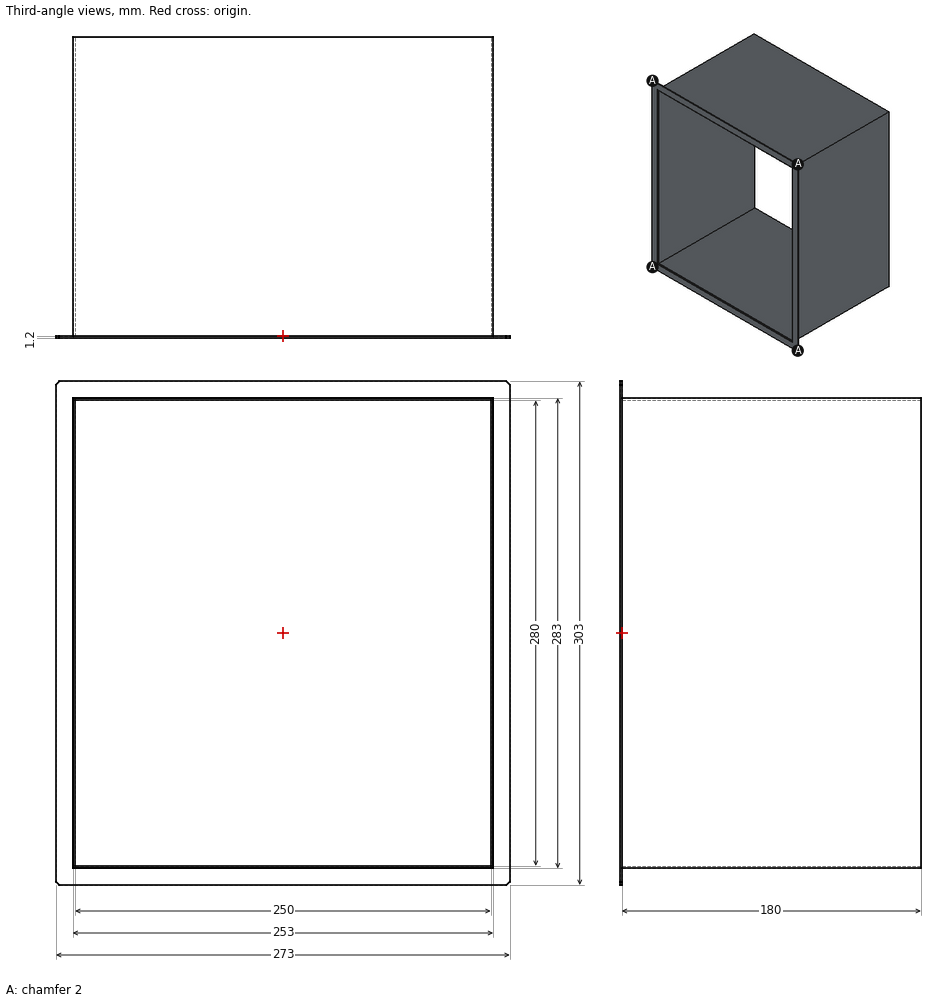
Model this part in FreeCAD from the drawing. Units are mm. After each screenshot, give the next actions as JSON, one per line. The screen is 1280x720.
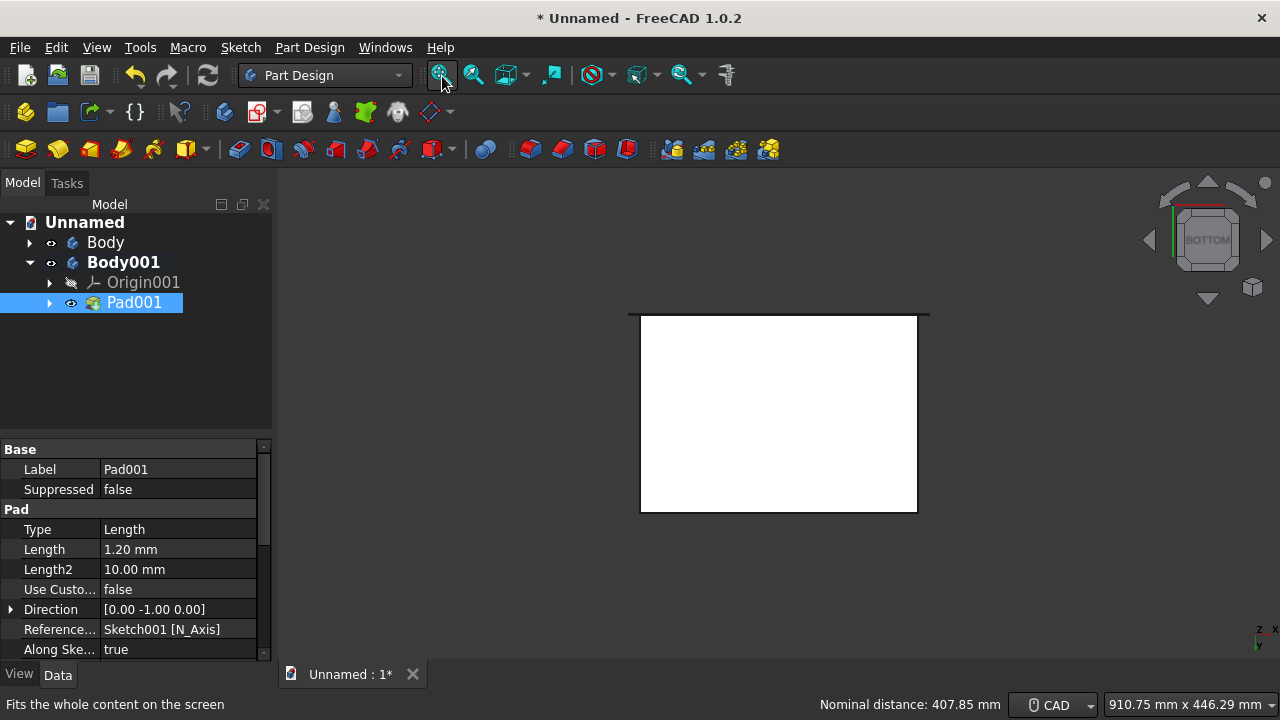
{"action": "scroll", "coordinate": [629, 313], "scroll_direction": "up", "scroll_amount": 15}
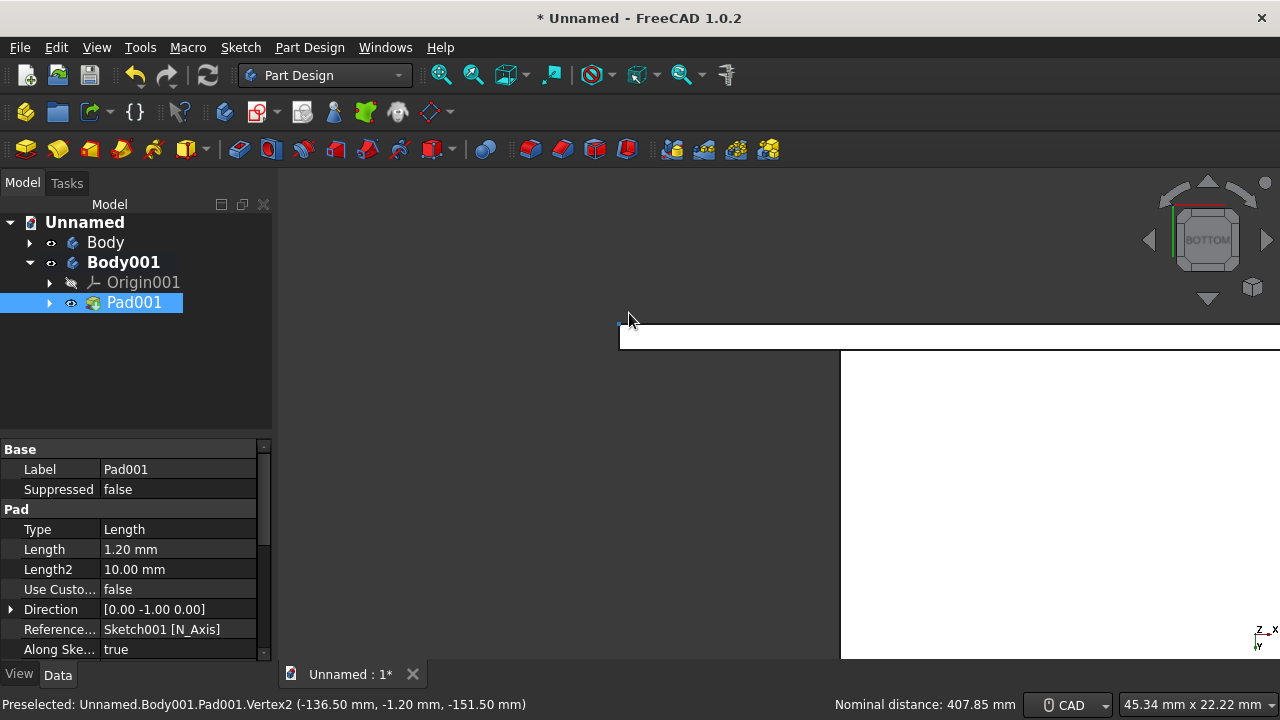
{"action": "left_click", "coordinate": [619, 336], "text": "ctrl"}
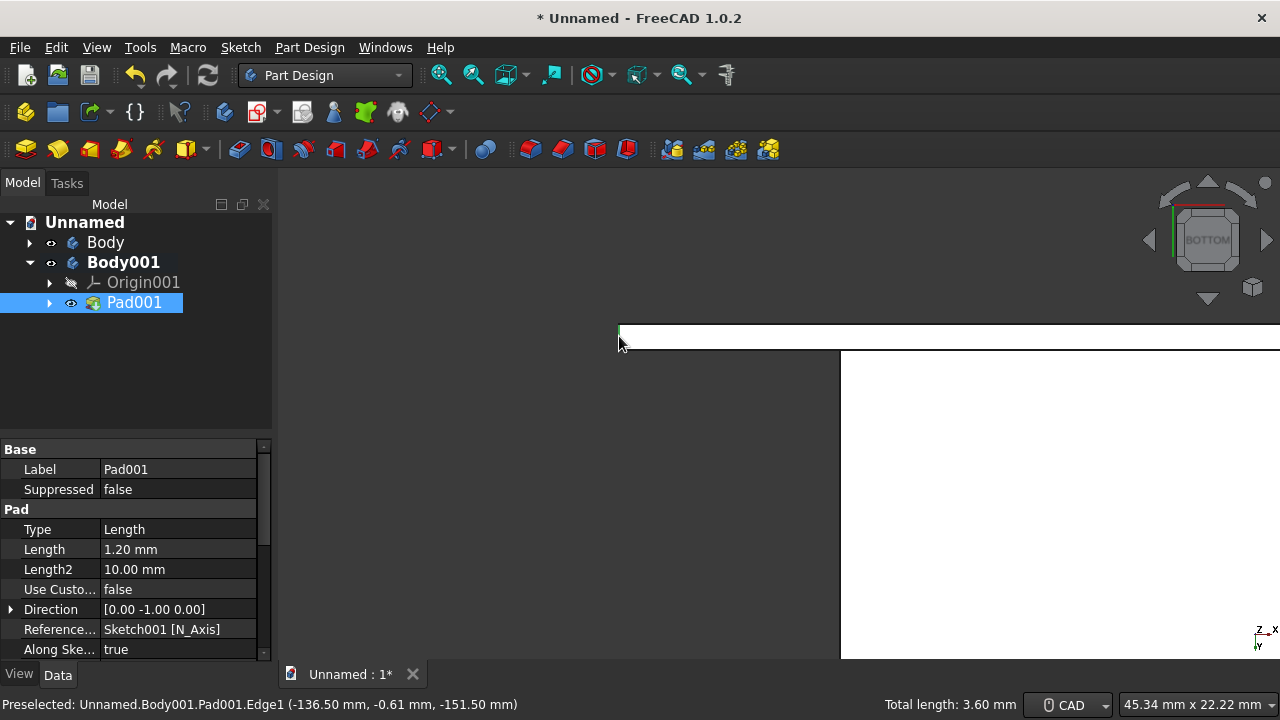
{"action": "key", "text": "v f"}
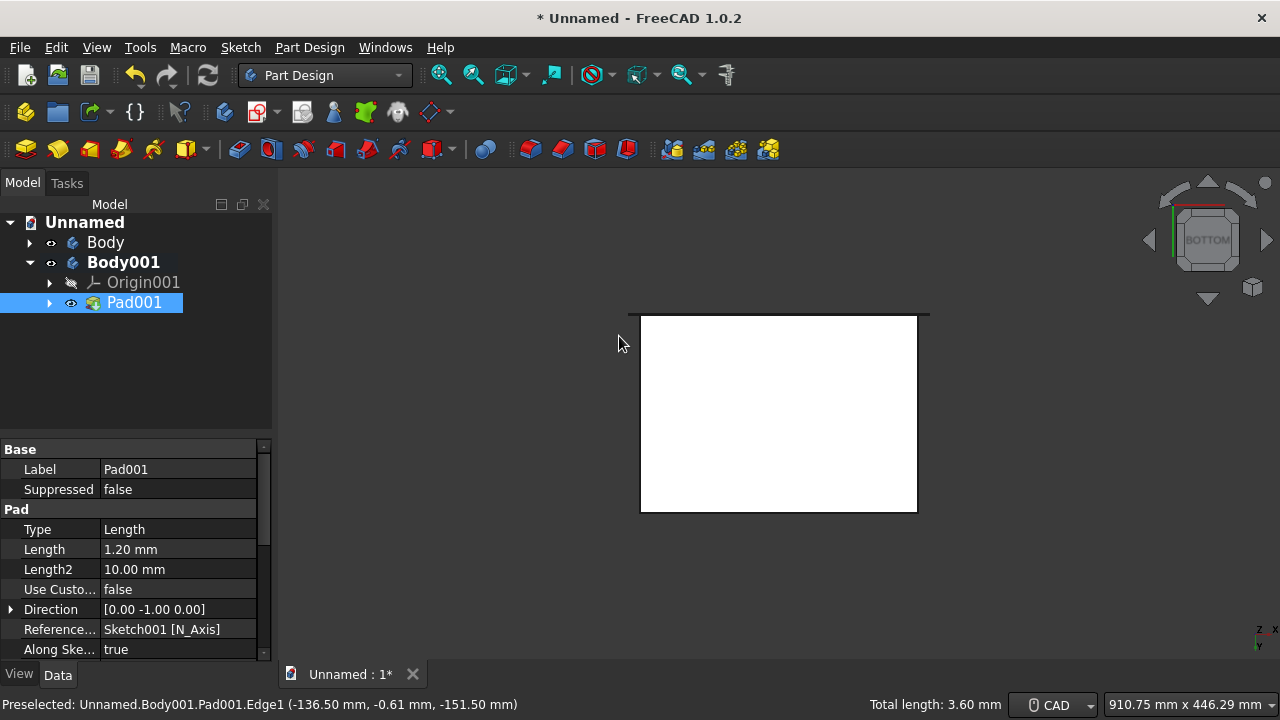
{"action": "key", "text": "4"}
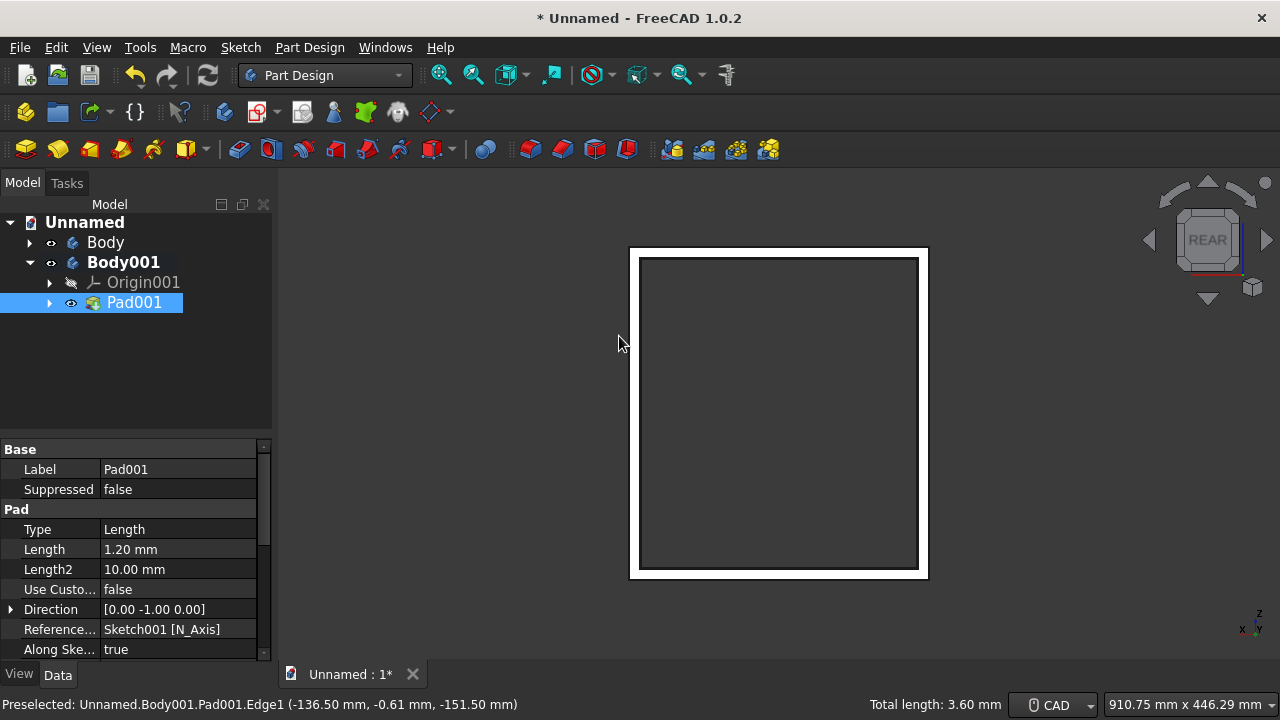
{"action": "scroll", "coordinate": [629, 246], "scroll_direction": "up", "scroll_amount": 15}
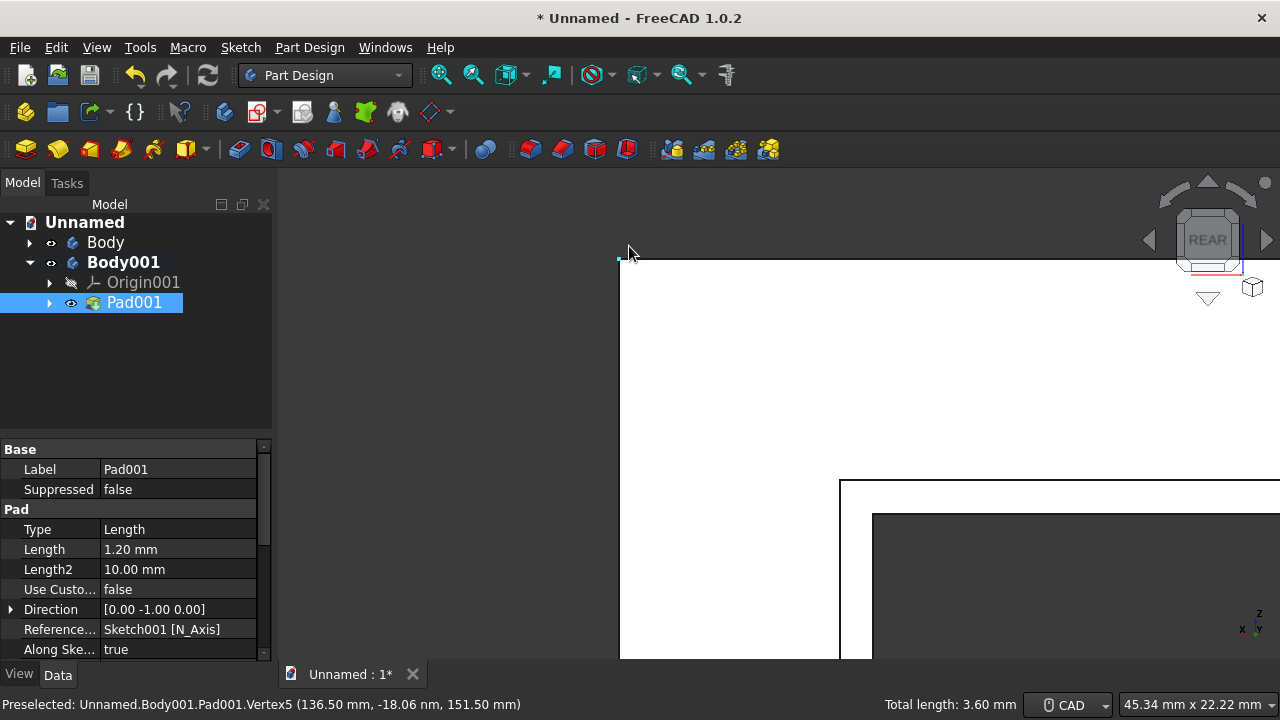
{"action": "key", "text": "v f"}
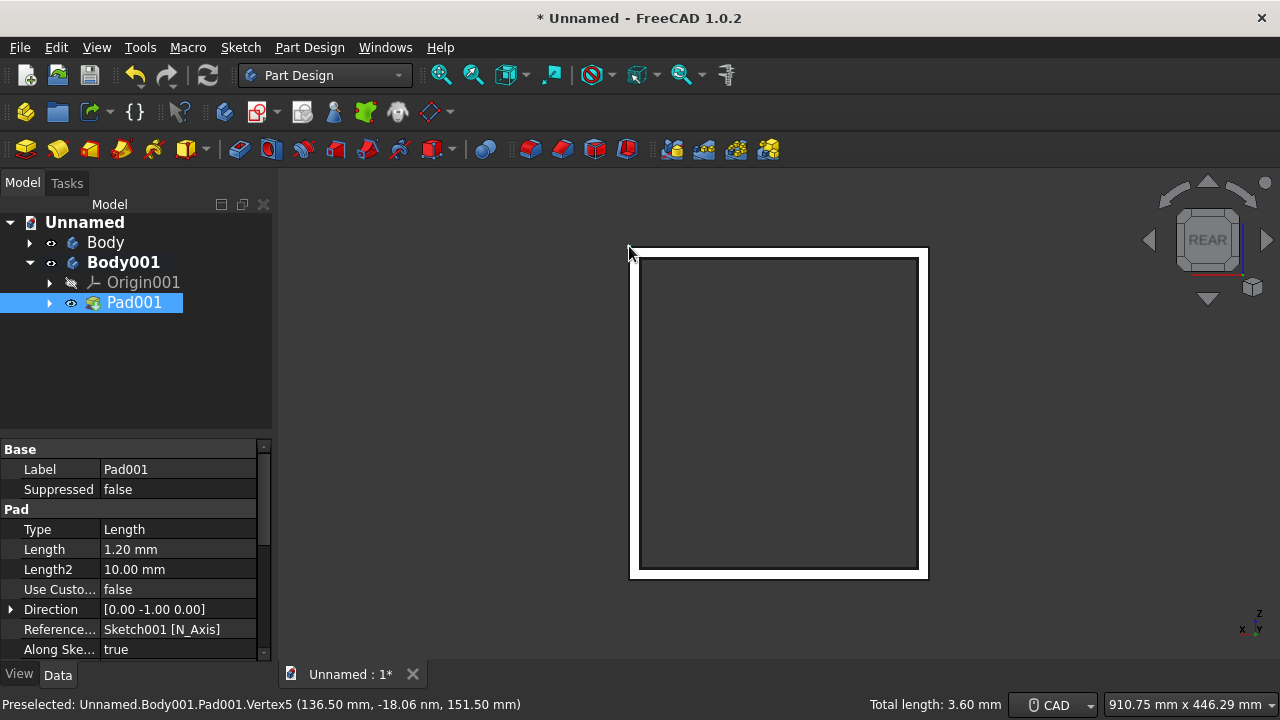
{"action": "key", "text": "6"}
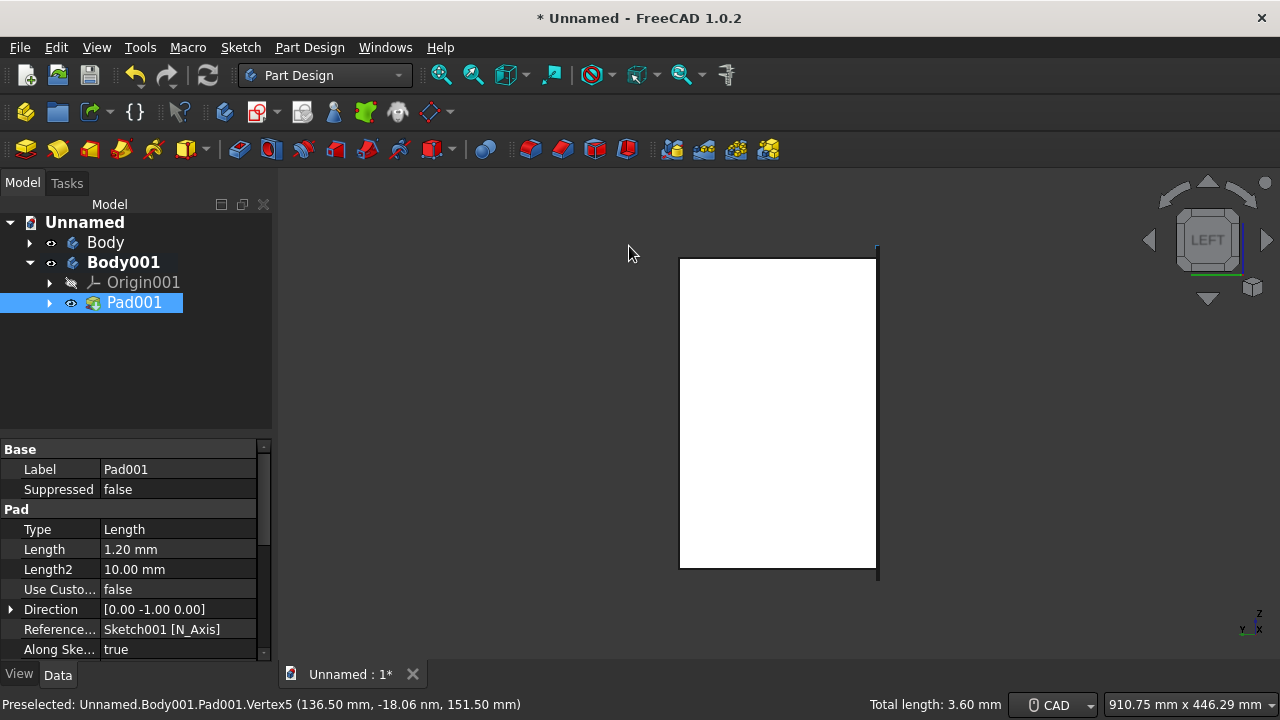
{"action": "scroll", "coordinate": [878, 246], "scroll_direction": "up", "scroll_amount": 15}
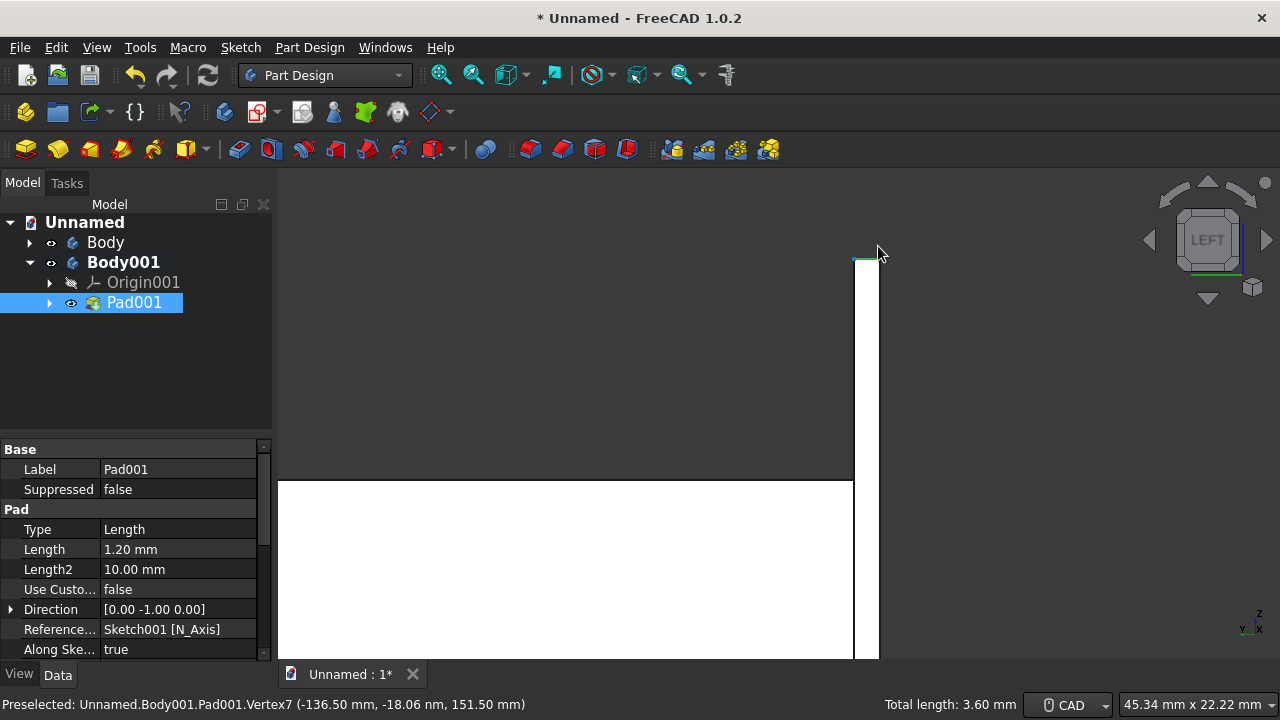
{"action": "left_click", "coordinate": [442, 76]}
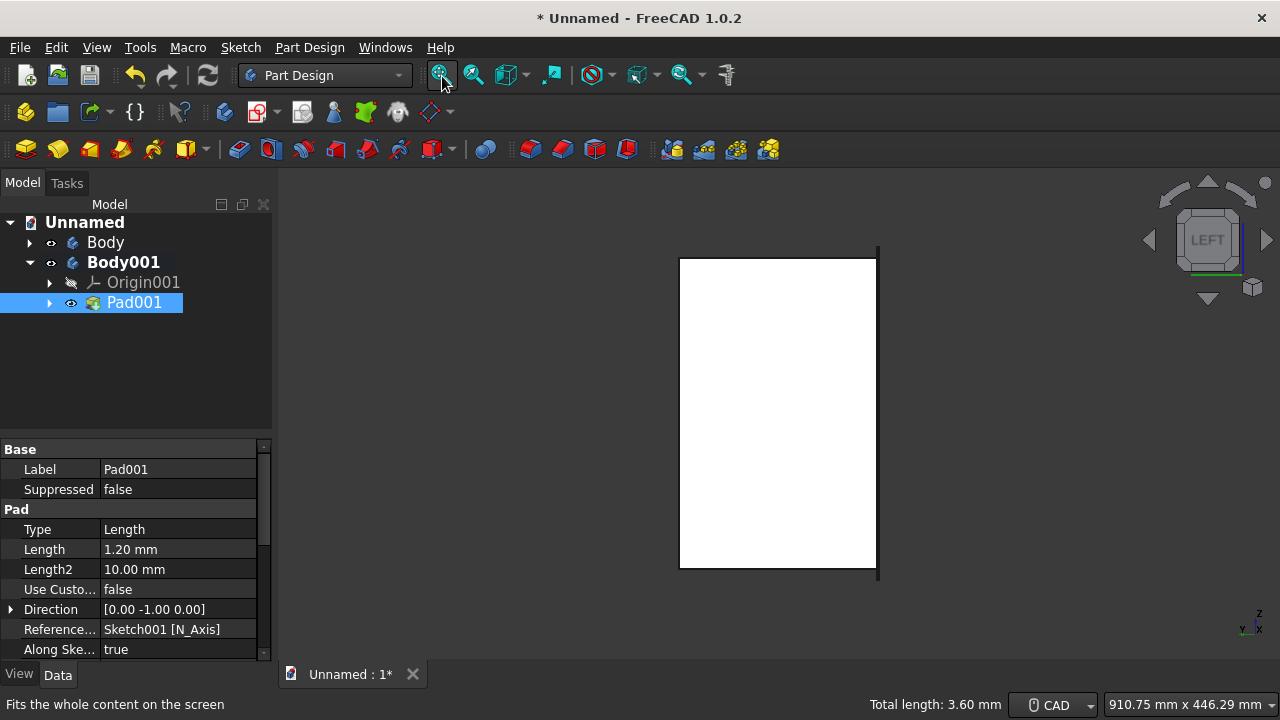
{"action": "key", "text": "v 3"}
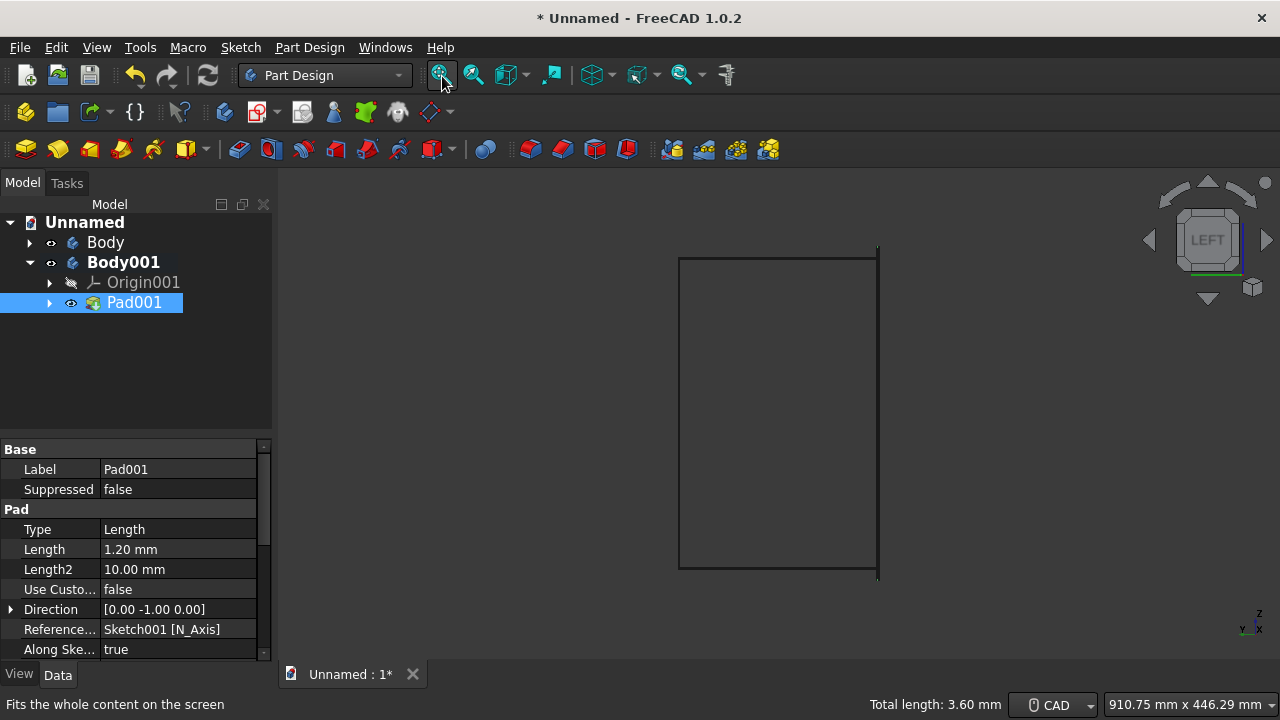
{"action": "key", "text": "0"}